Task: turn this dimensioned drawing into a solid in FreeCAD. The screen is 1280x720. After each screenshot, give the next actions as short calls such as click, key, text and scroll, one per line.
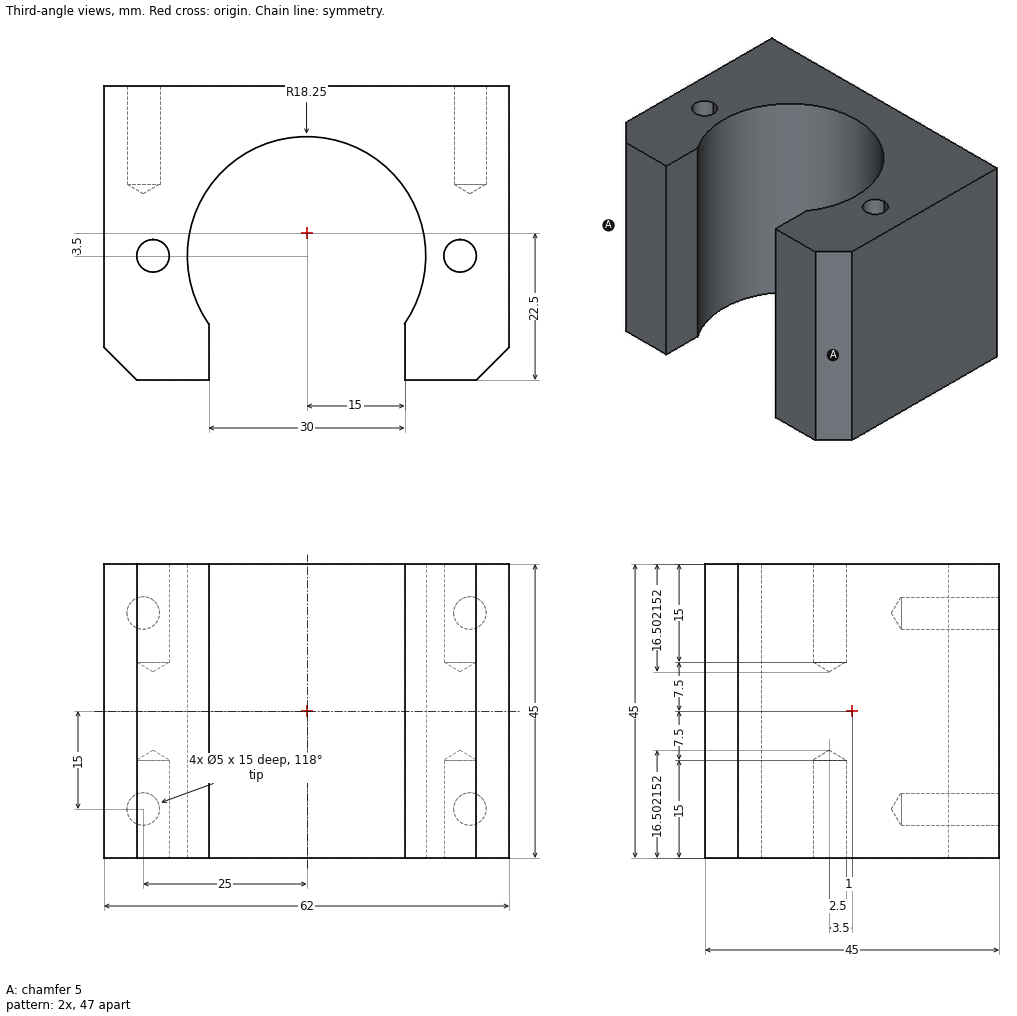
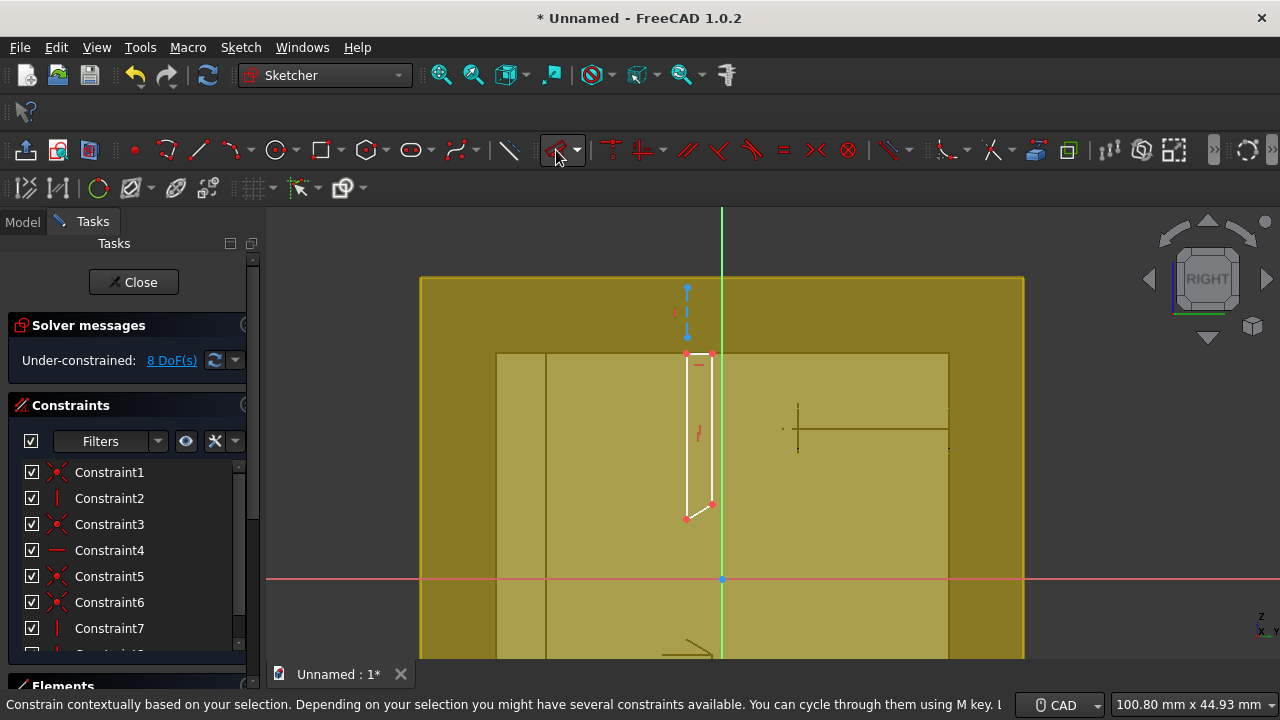
scroll(712, 459, up, 2)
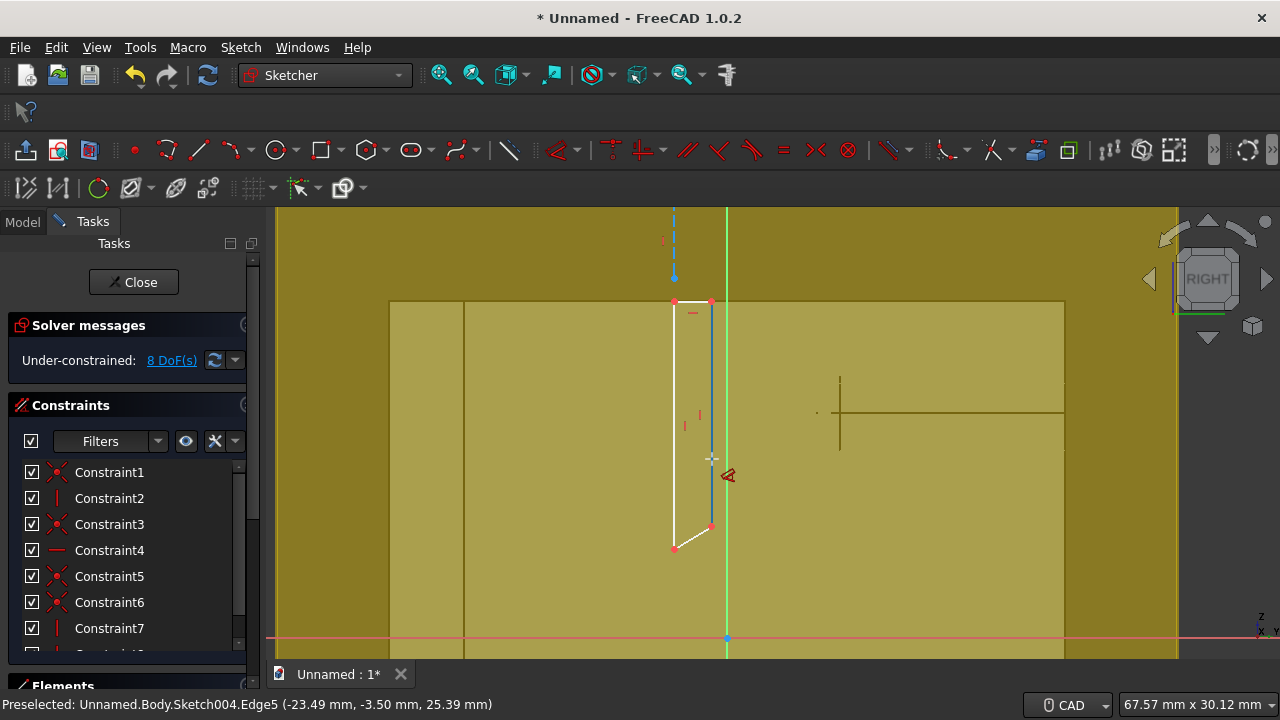
click(712, 459)
click(746, 414)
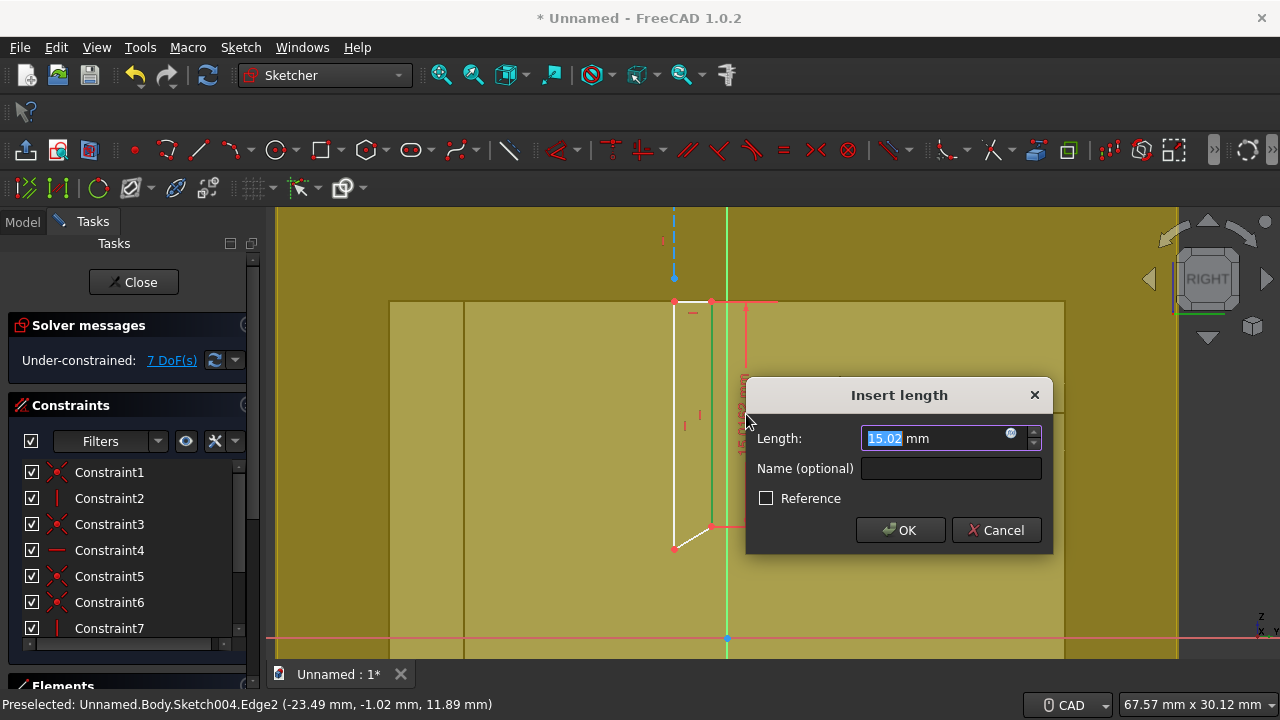
text(15)
key(Return)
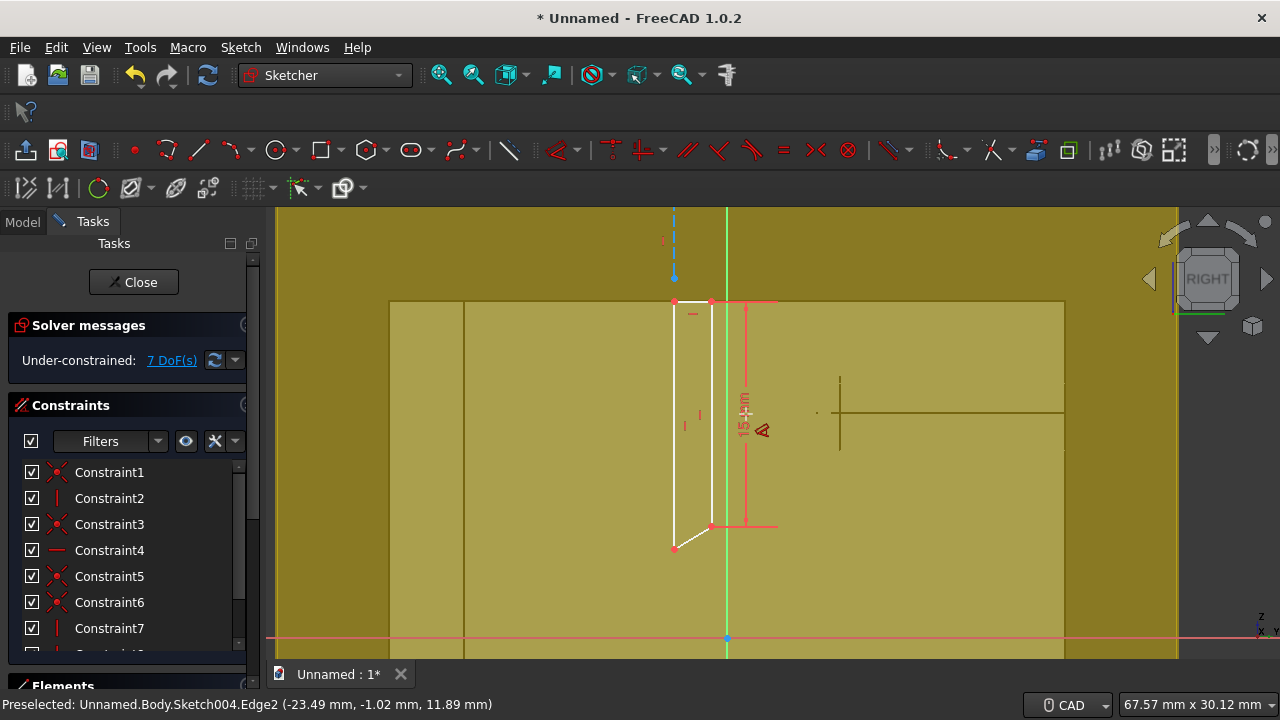
scroll(712, 527, up, 5)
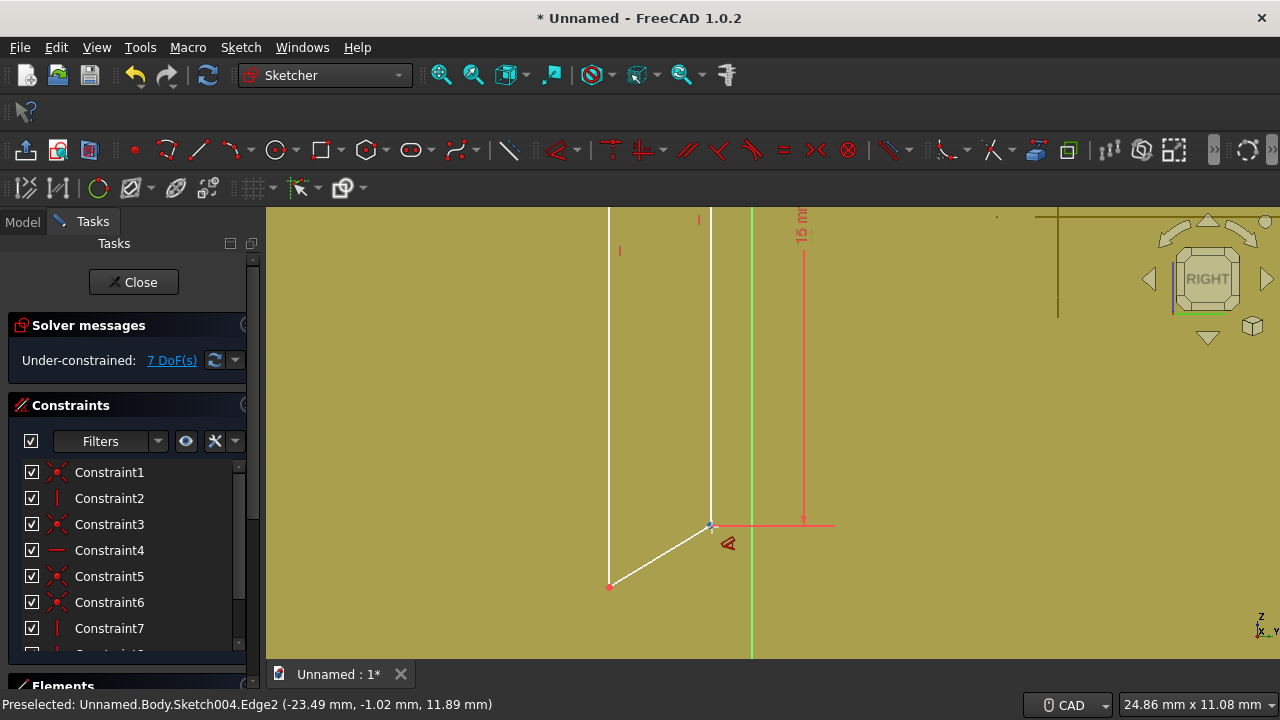
click(711, 526)
click(731, 492)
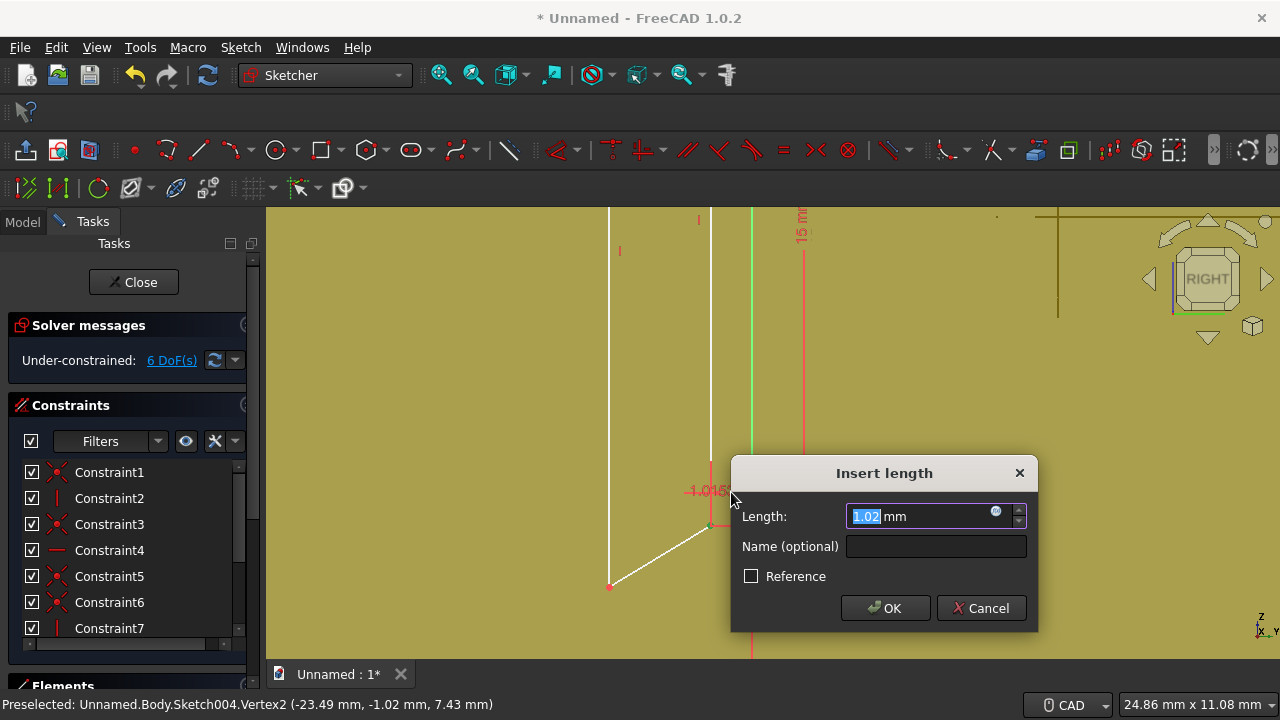
text(1)
key(Return)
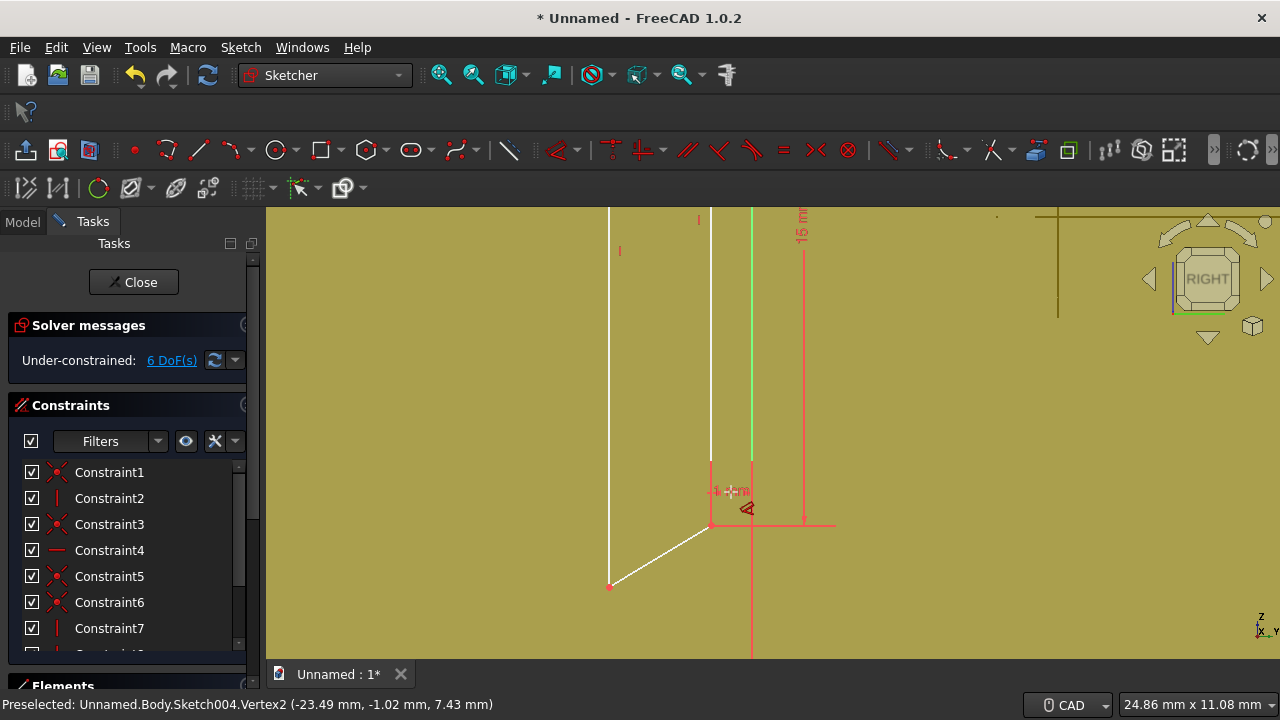
scroll(712, 498, down, 7)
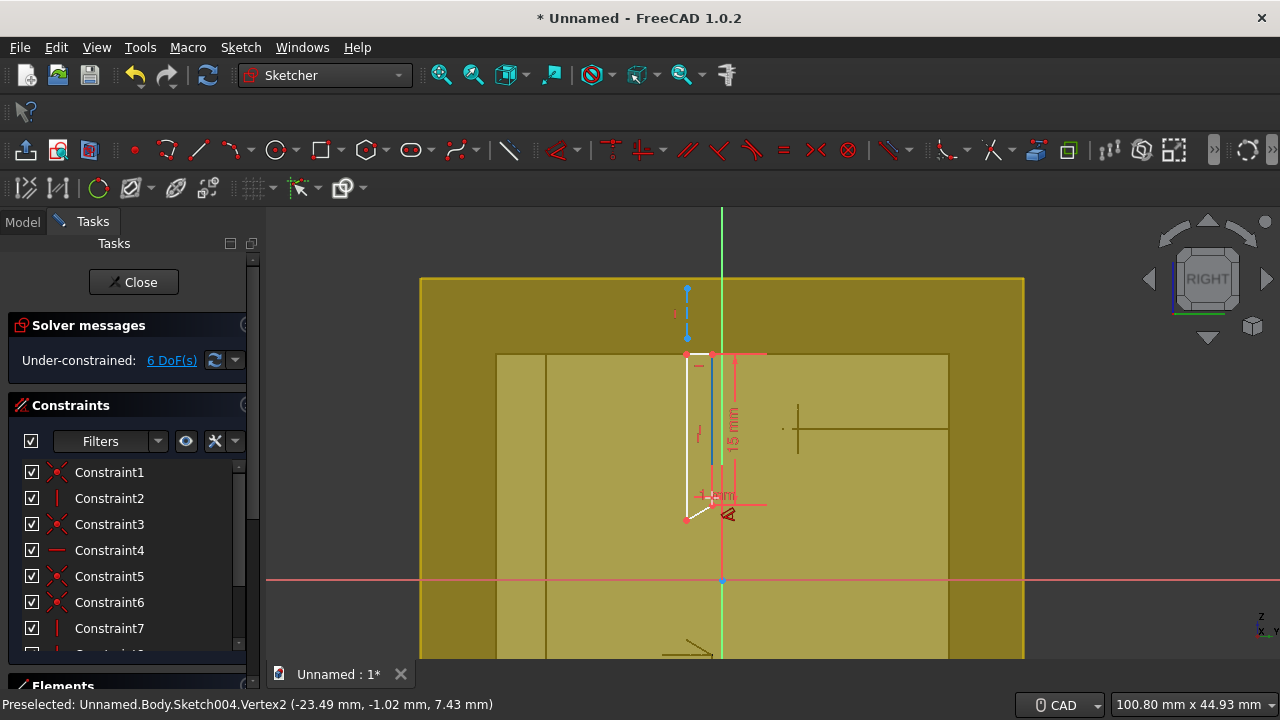
scroll(705, 354, up, 4)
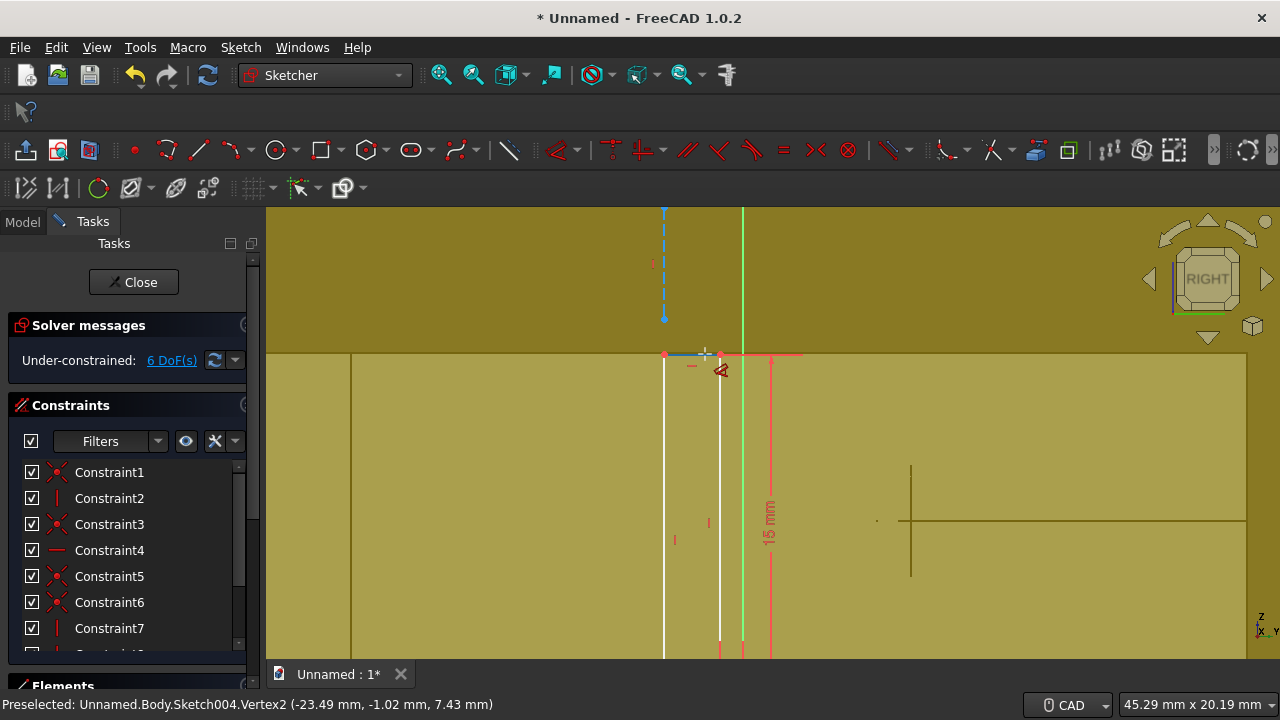
click(704, 355)
click(692, 321)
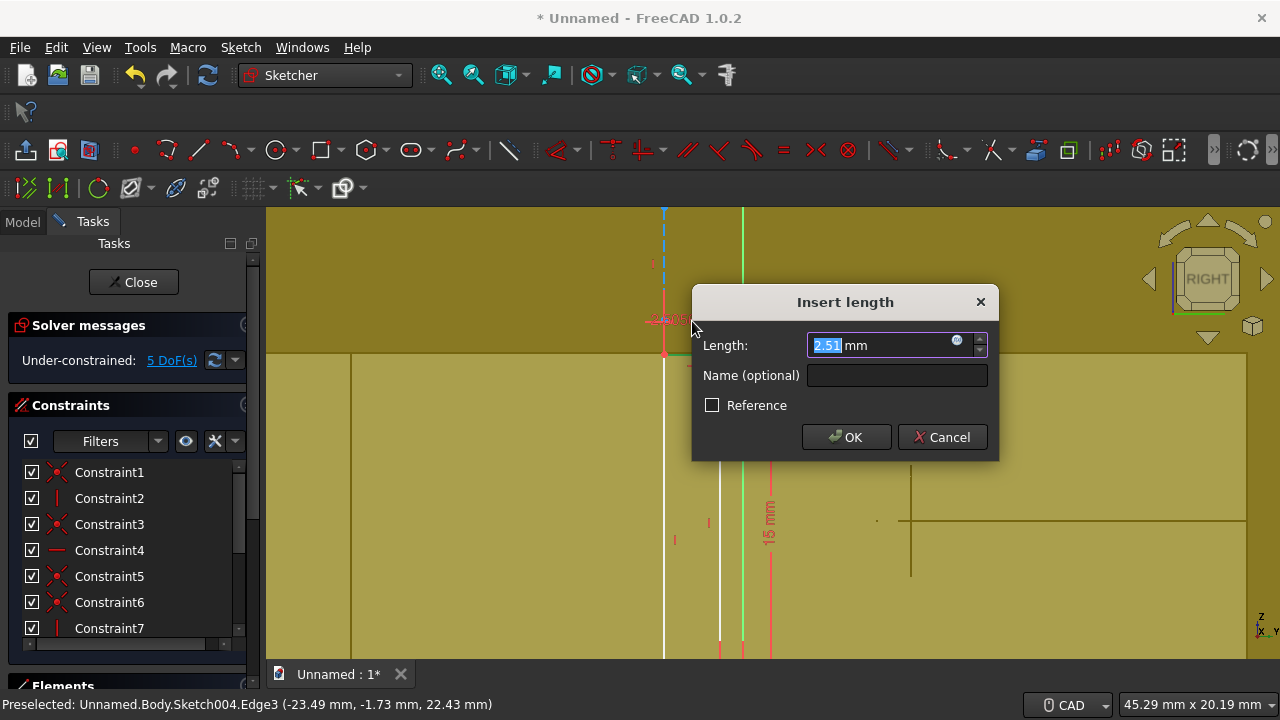
text(2.5)
key(Return)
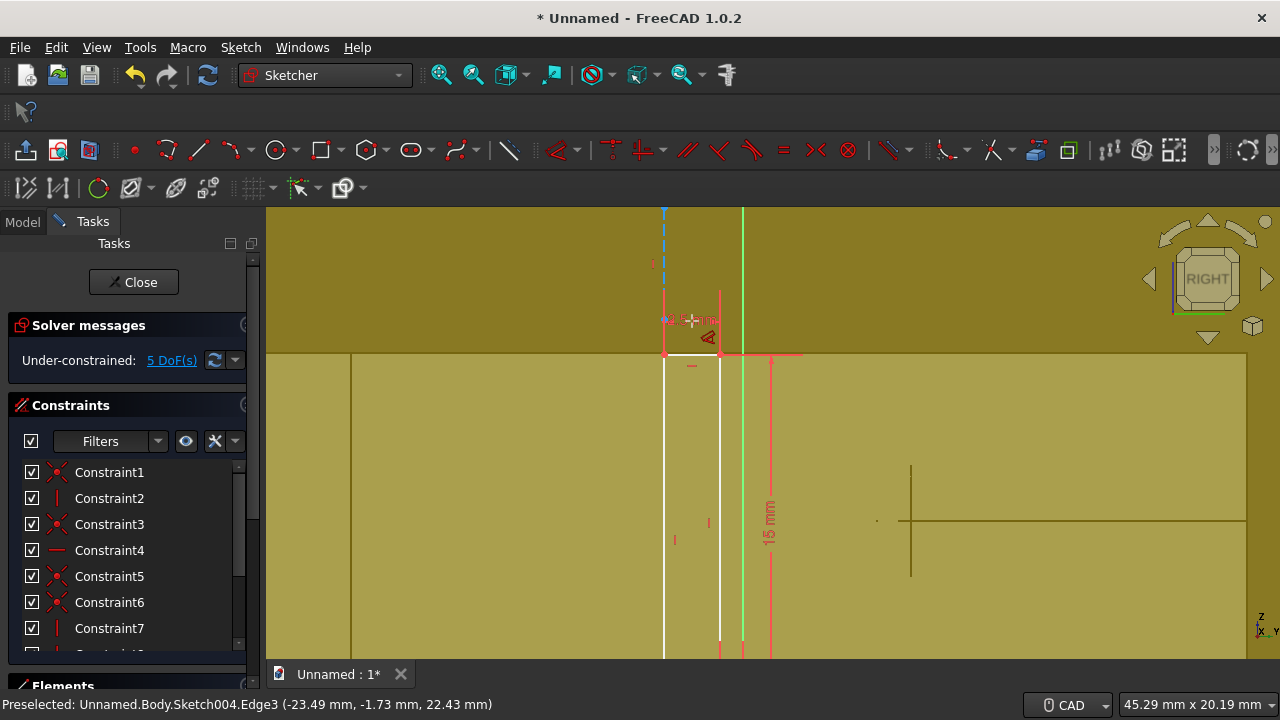
scroll(705, 353, down, 4)